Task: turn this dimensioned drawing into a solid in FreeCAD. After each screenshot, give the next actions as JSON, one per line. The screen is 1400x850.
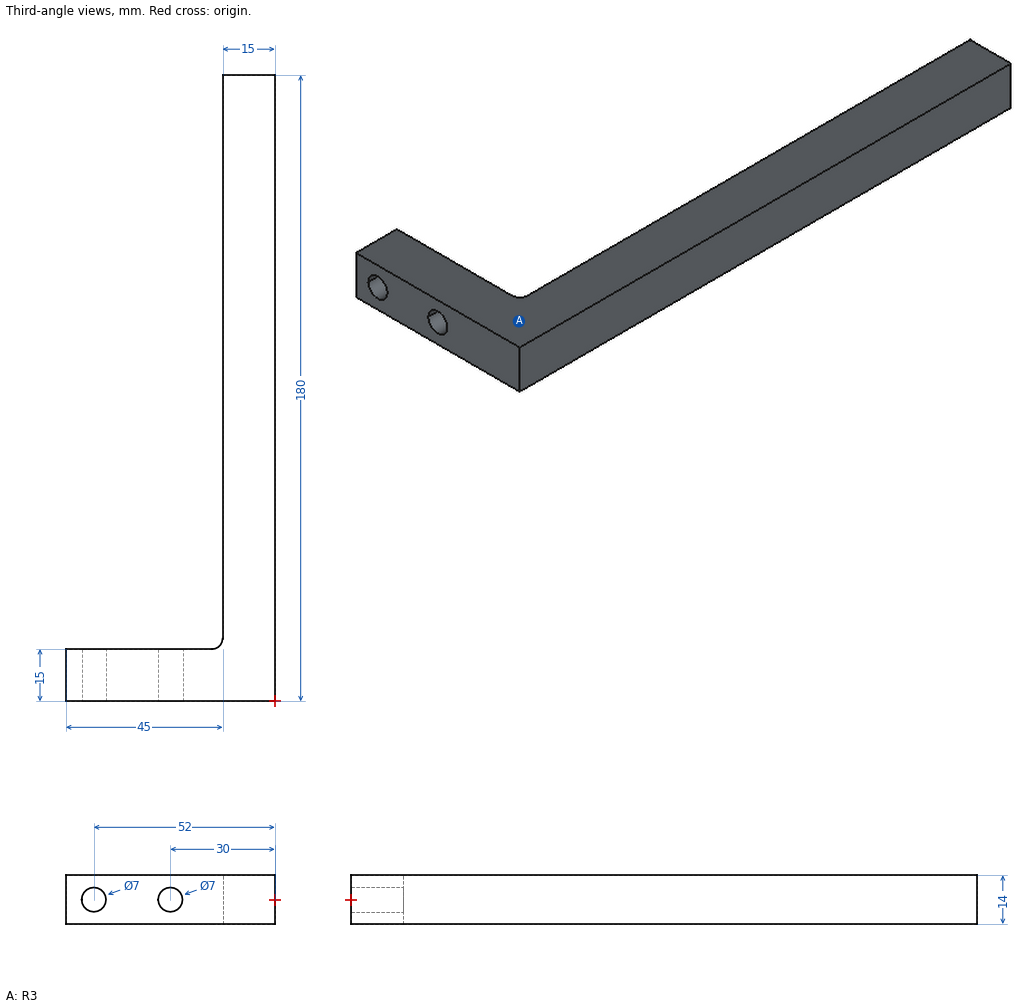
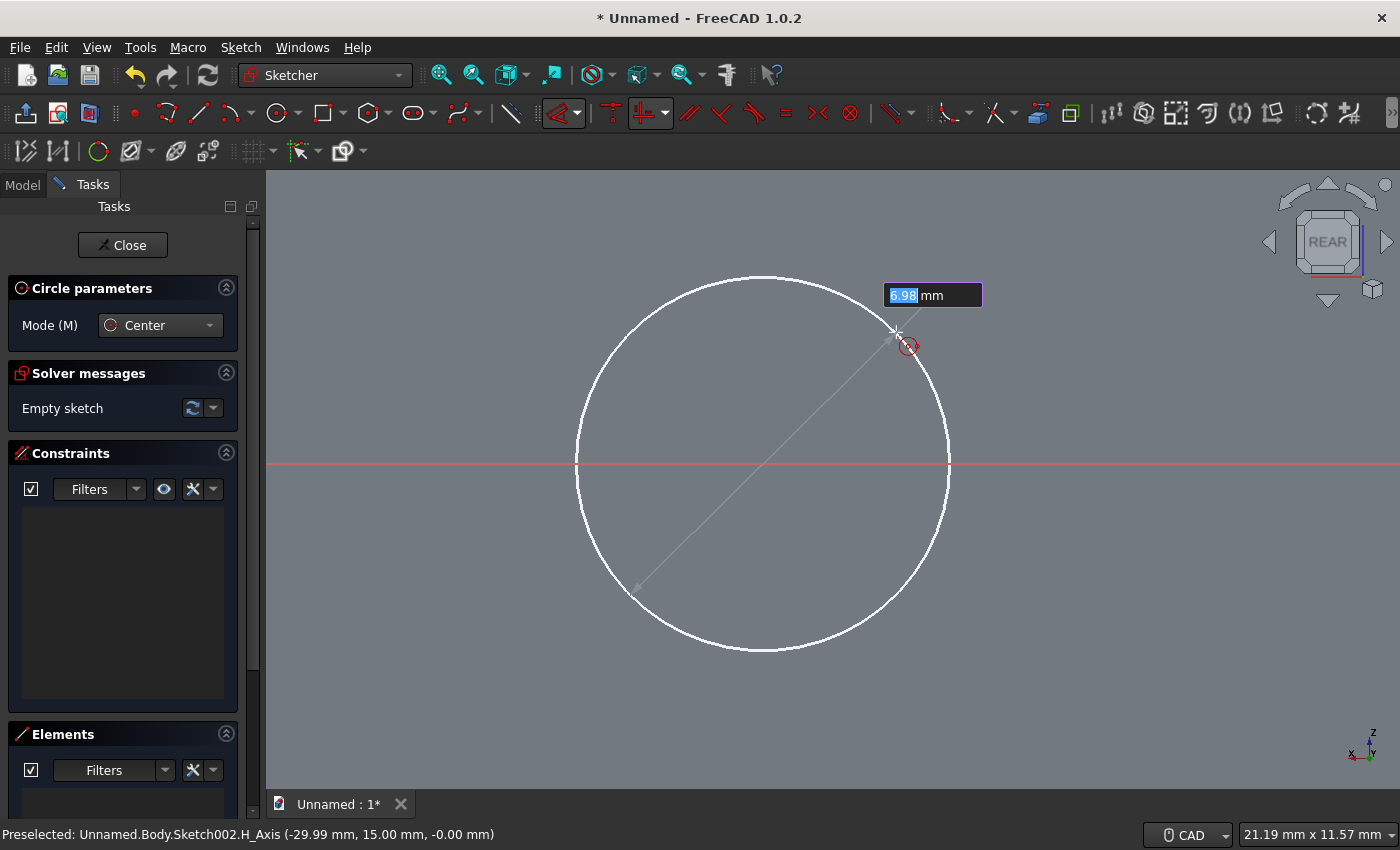
{"action": "type", "text": "7"}
{"action": "key", "text": "Return"}
{"action": "key", "text": "Escape"}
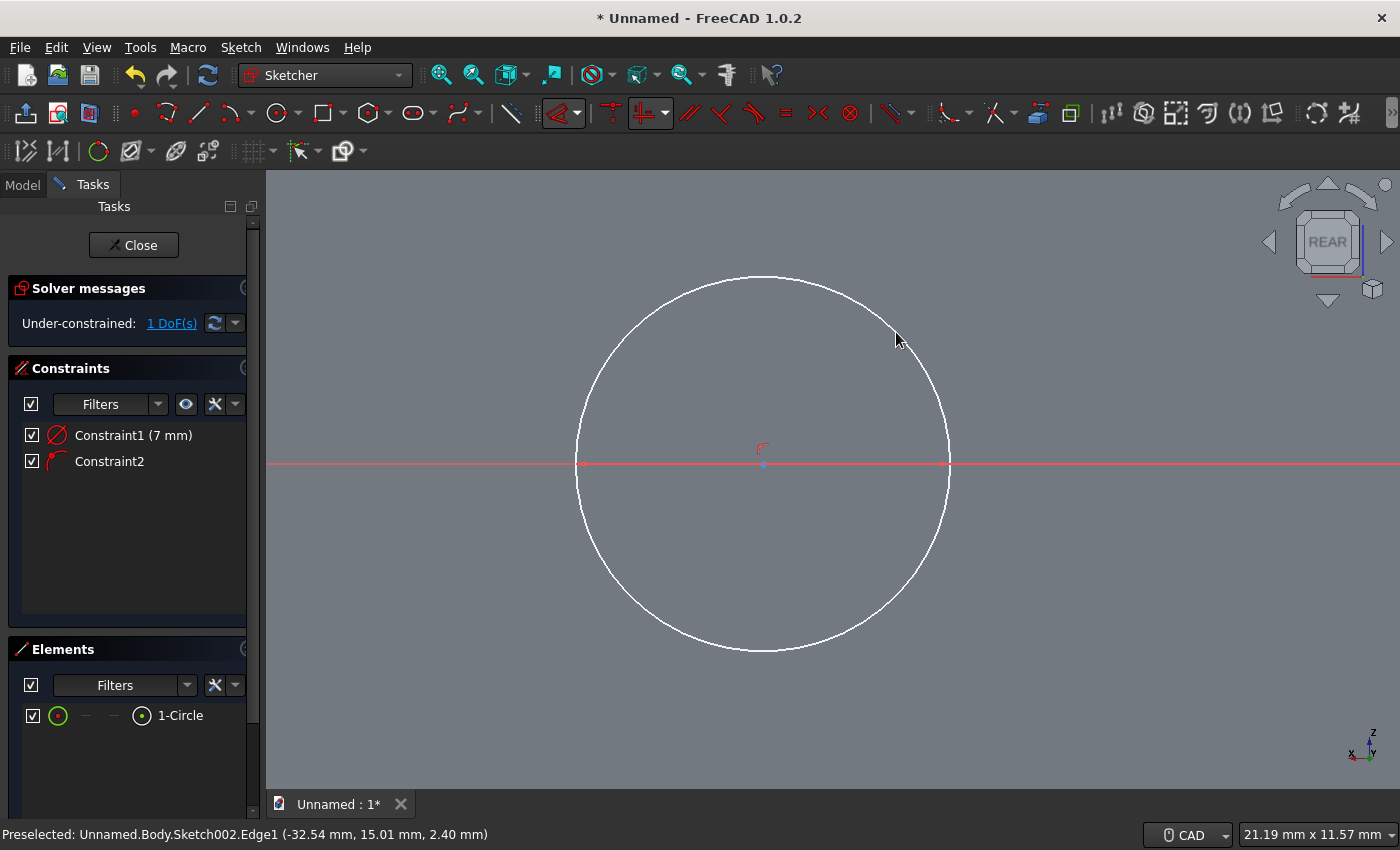
{"action": "left_click", "coordinate": [763, 464]}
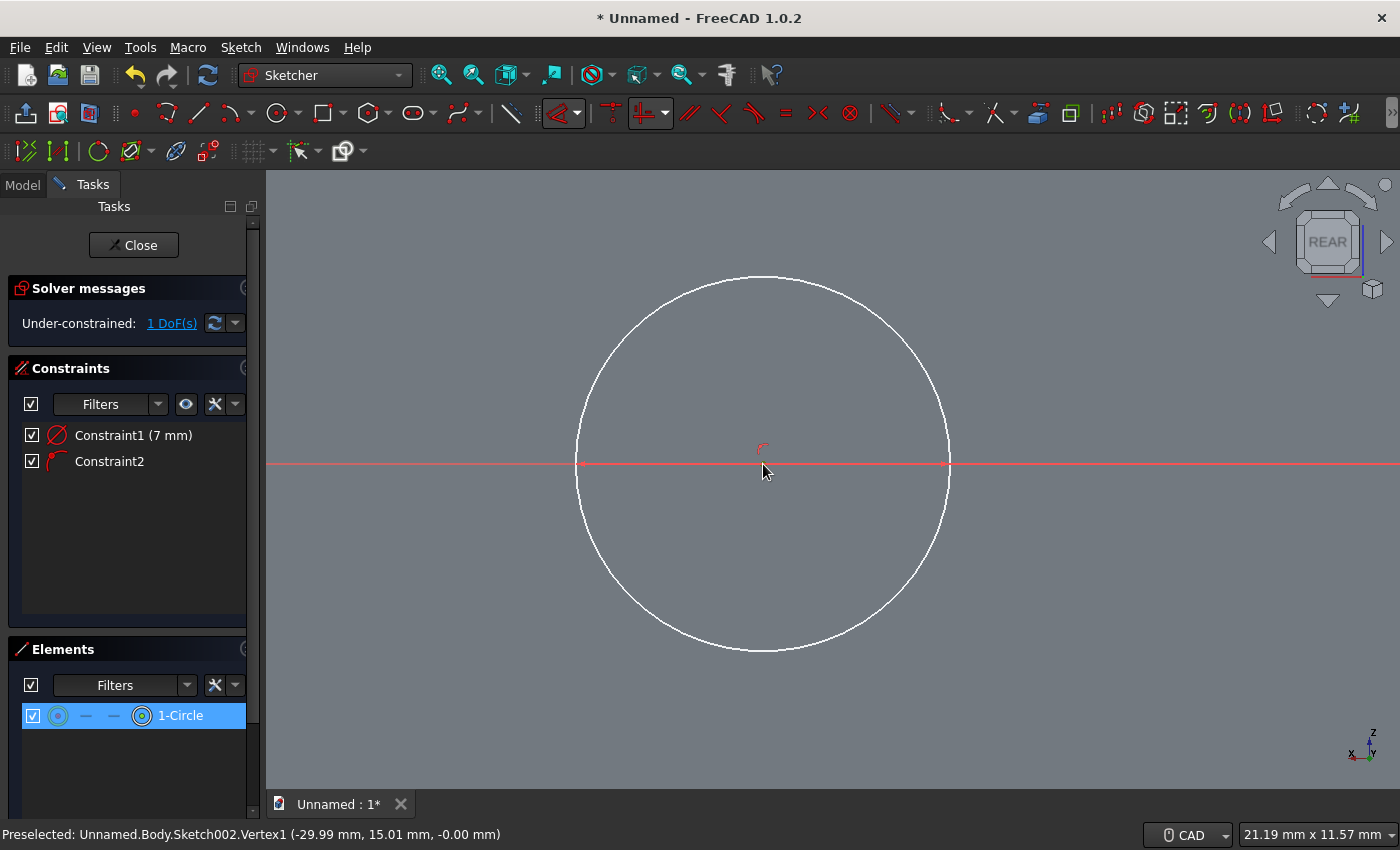
{"action": "key", "text": "l"}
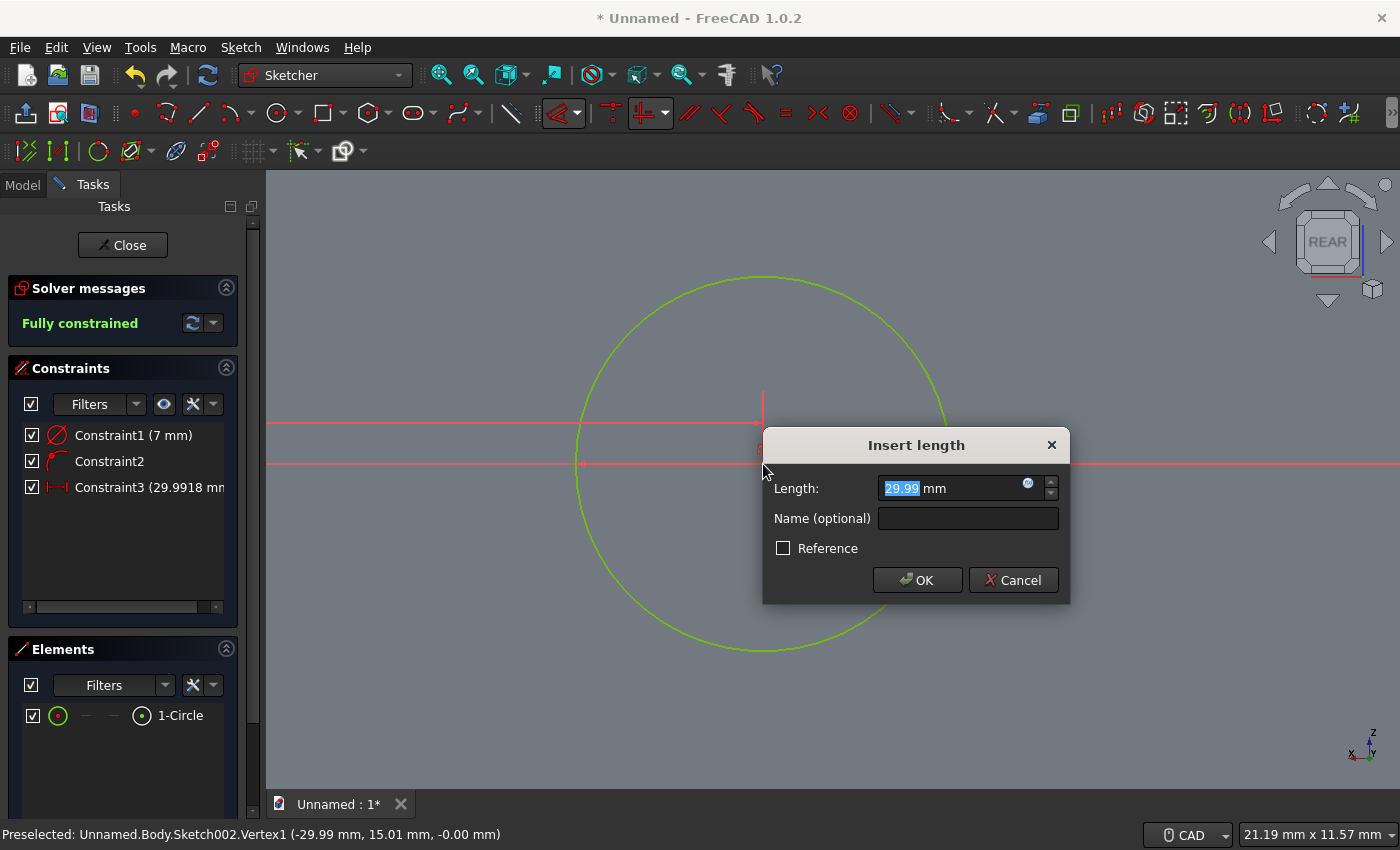
{"action": "type", "text": "30"}
{"action": "key", "text": "Return"}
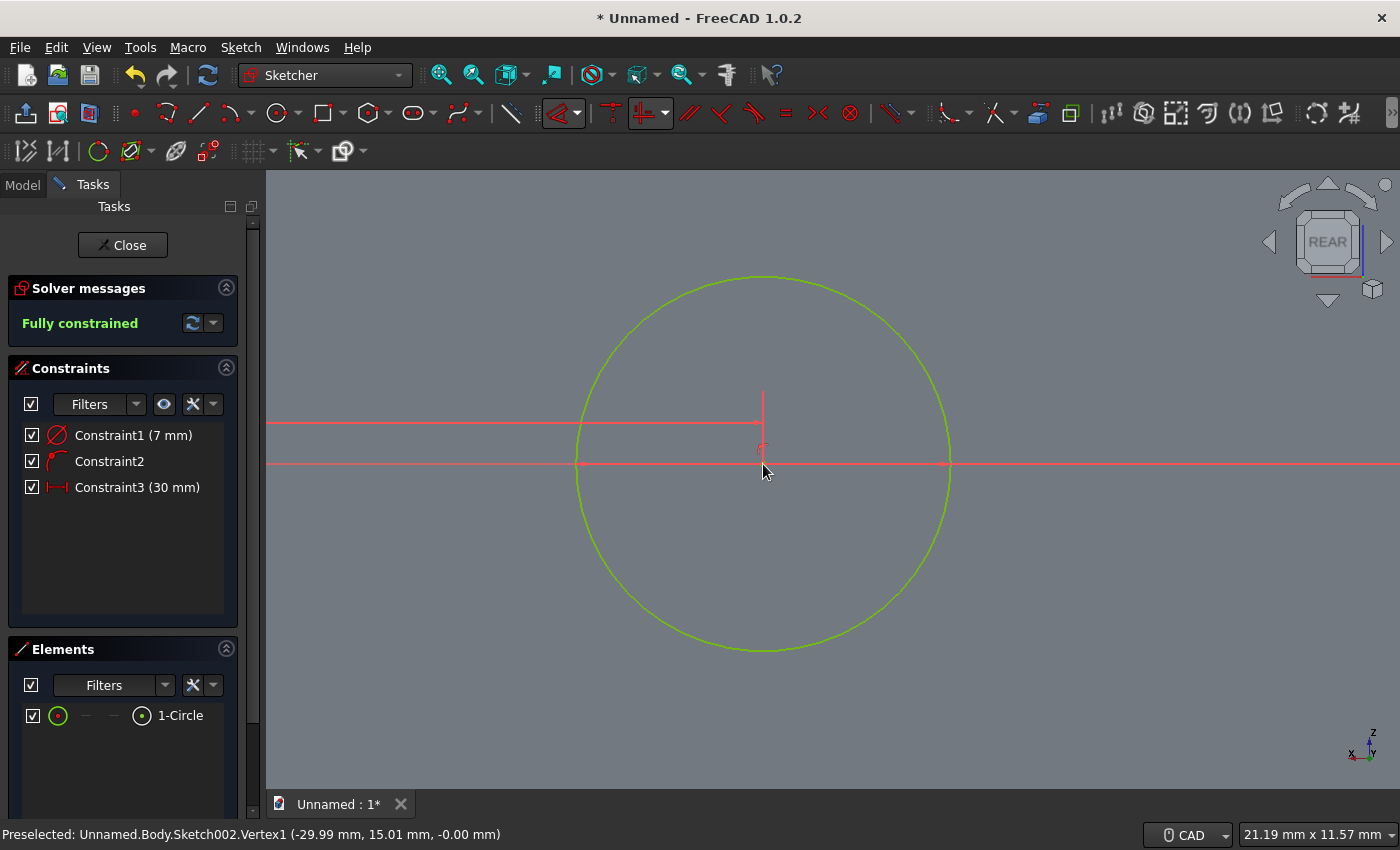
{"action": "left_click", "coordinate": [123, 245]}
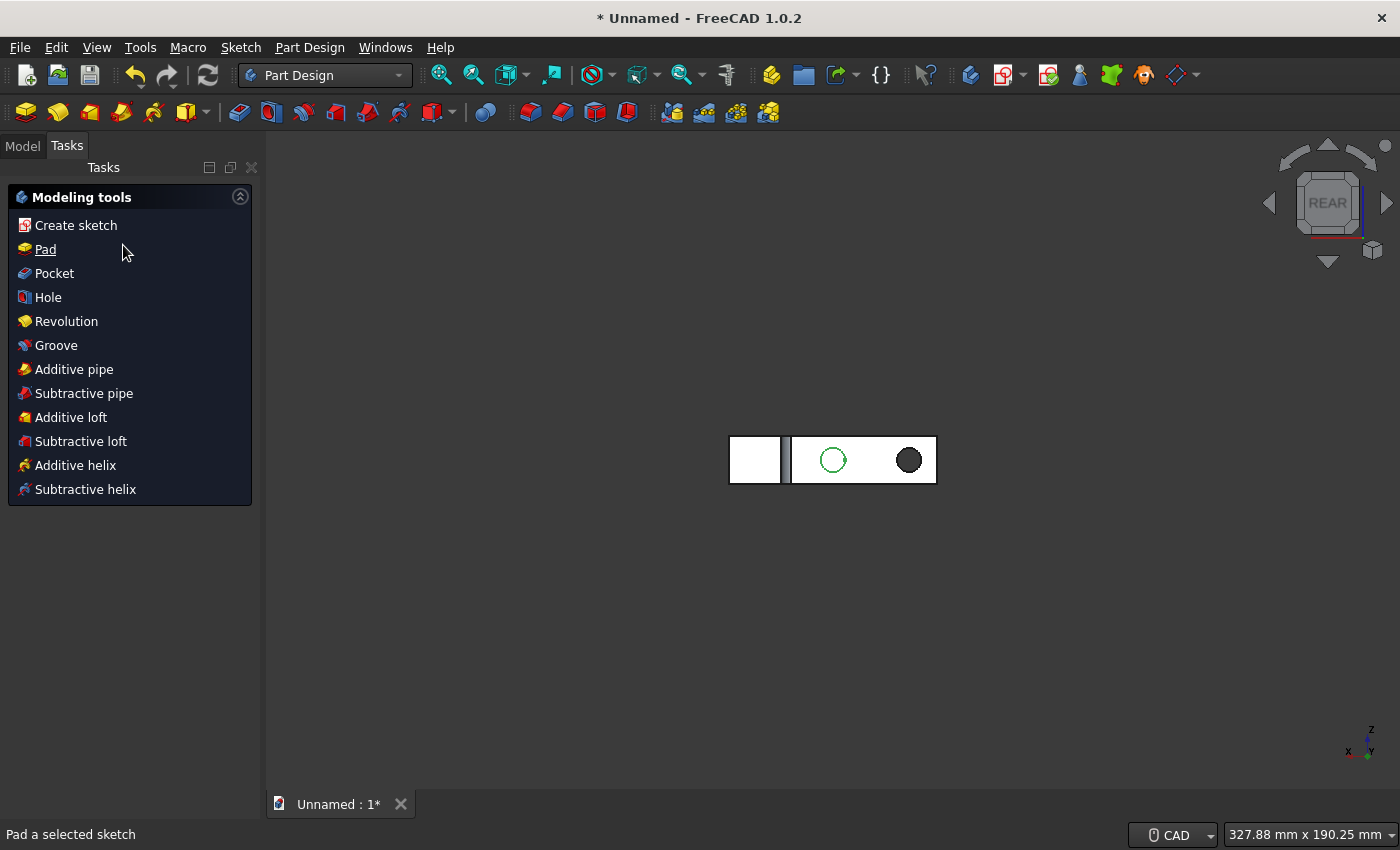
{"action": "left_click", "coordinate": [240, 112]}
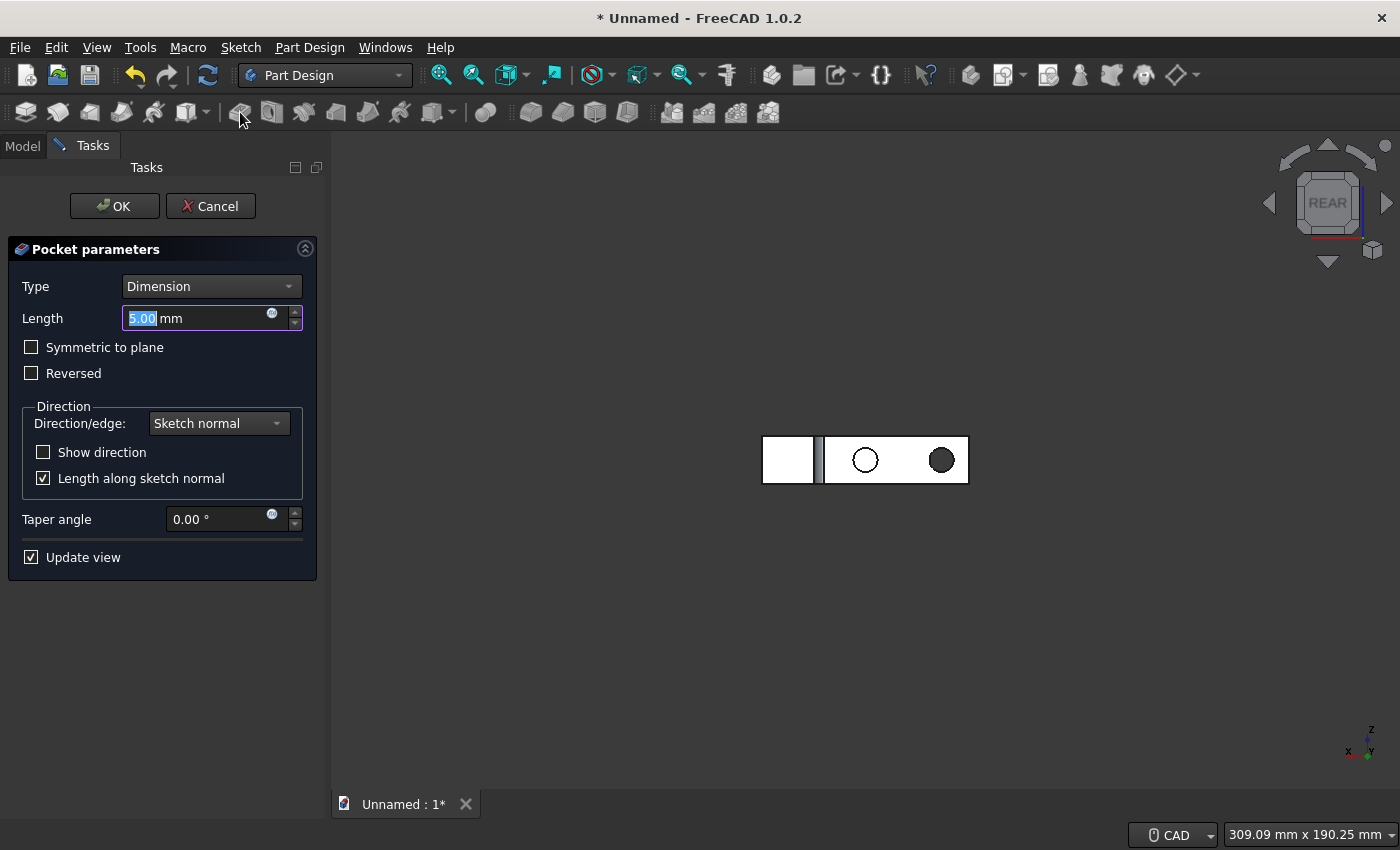
{"action": "left_click", "coordinate": [212, 286]}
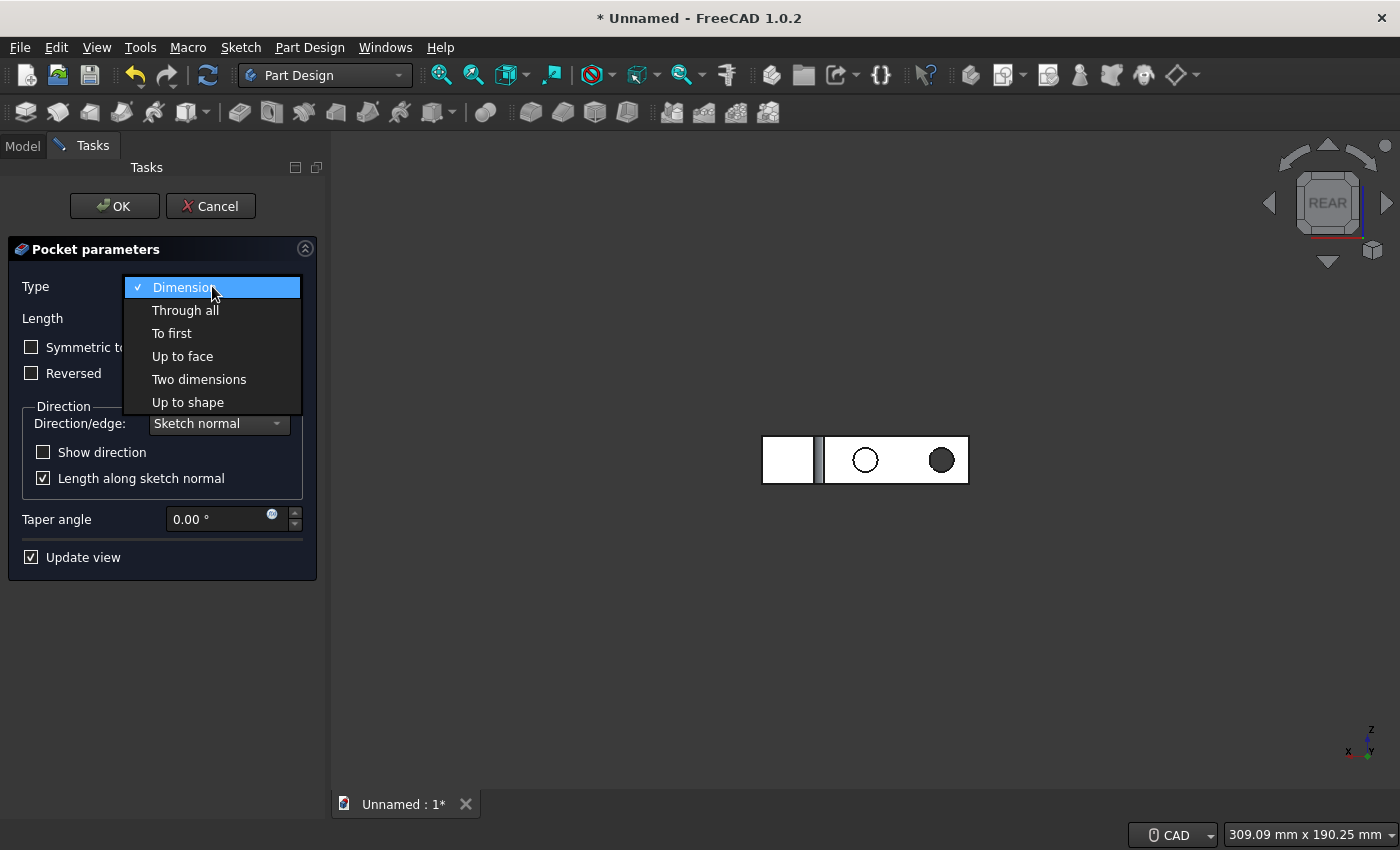
{"action": "left_click", "coordinate": [212, 334]}